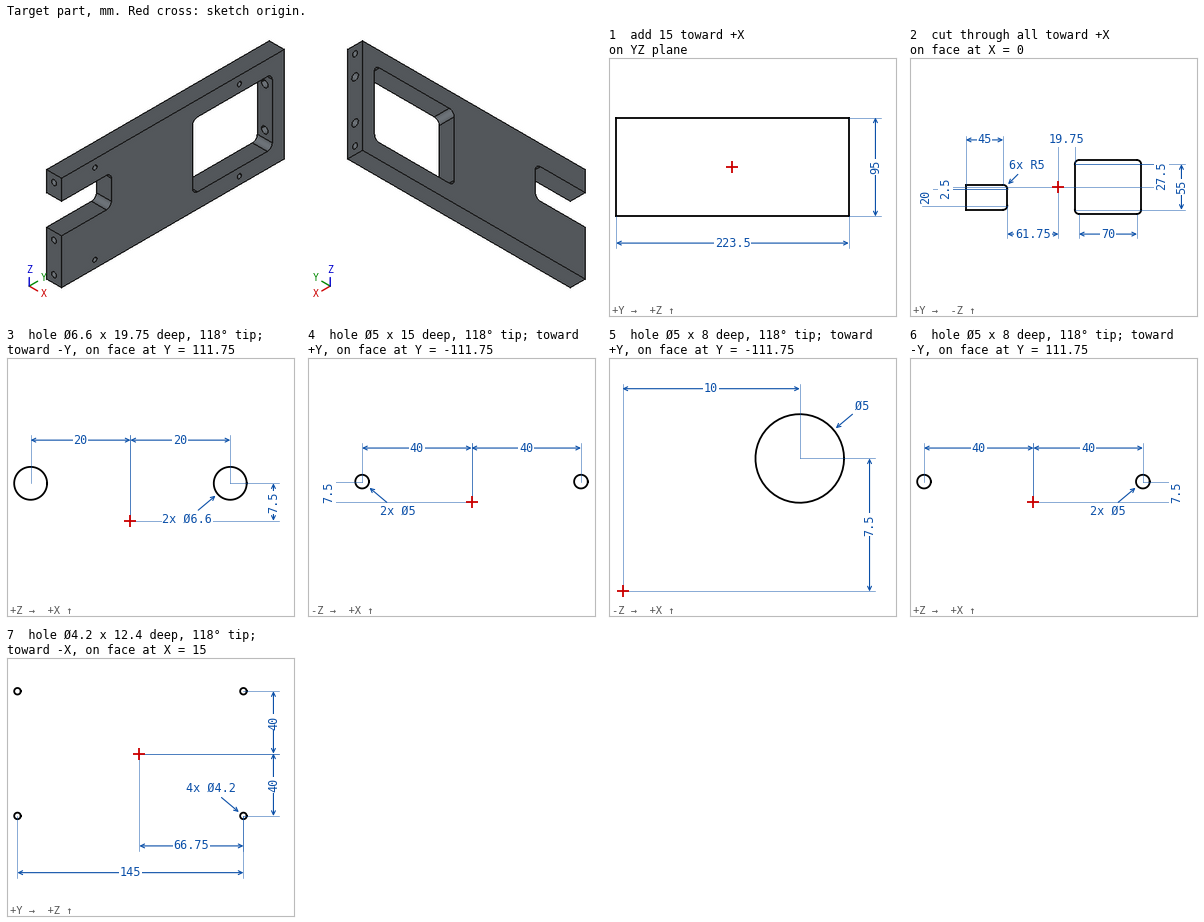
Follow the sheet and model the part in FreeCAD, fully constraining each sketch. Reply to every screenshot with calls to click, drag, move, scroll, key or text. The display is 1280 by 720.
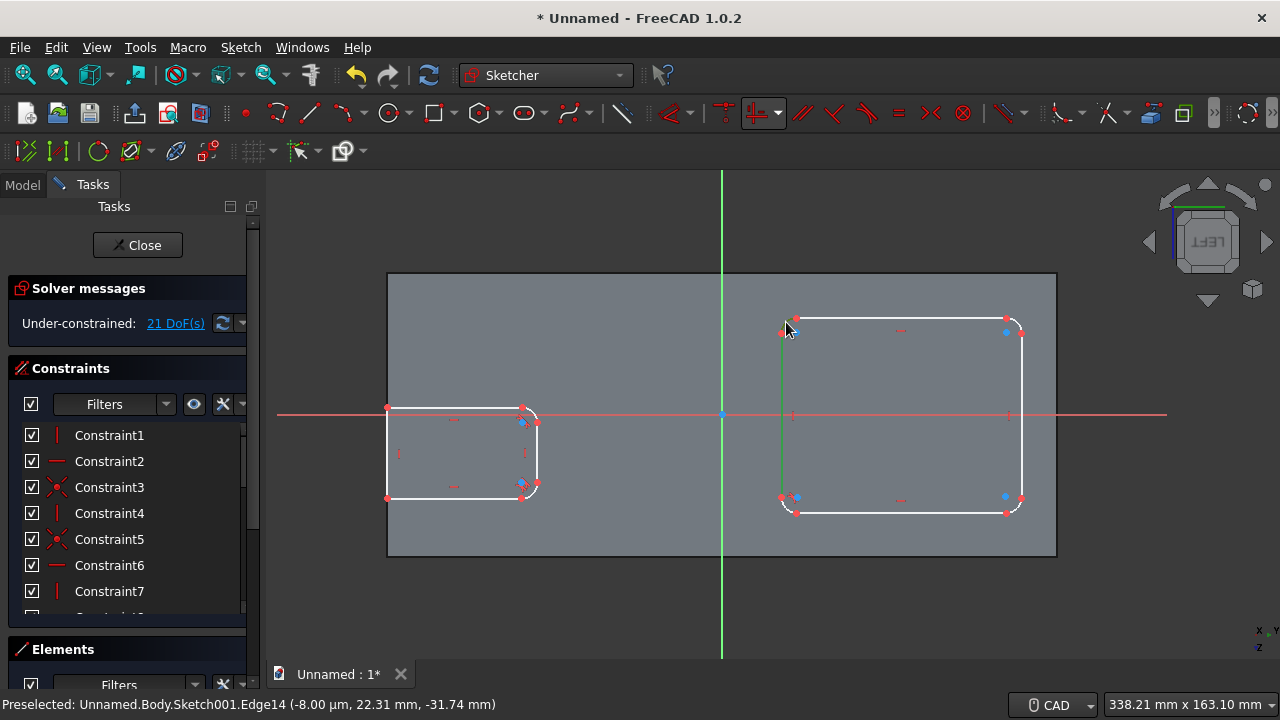
click(868, 114)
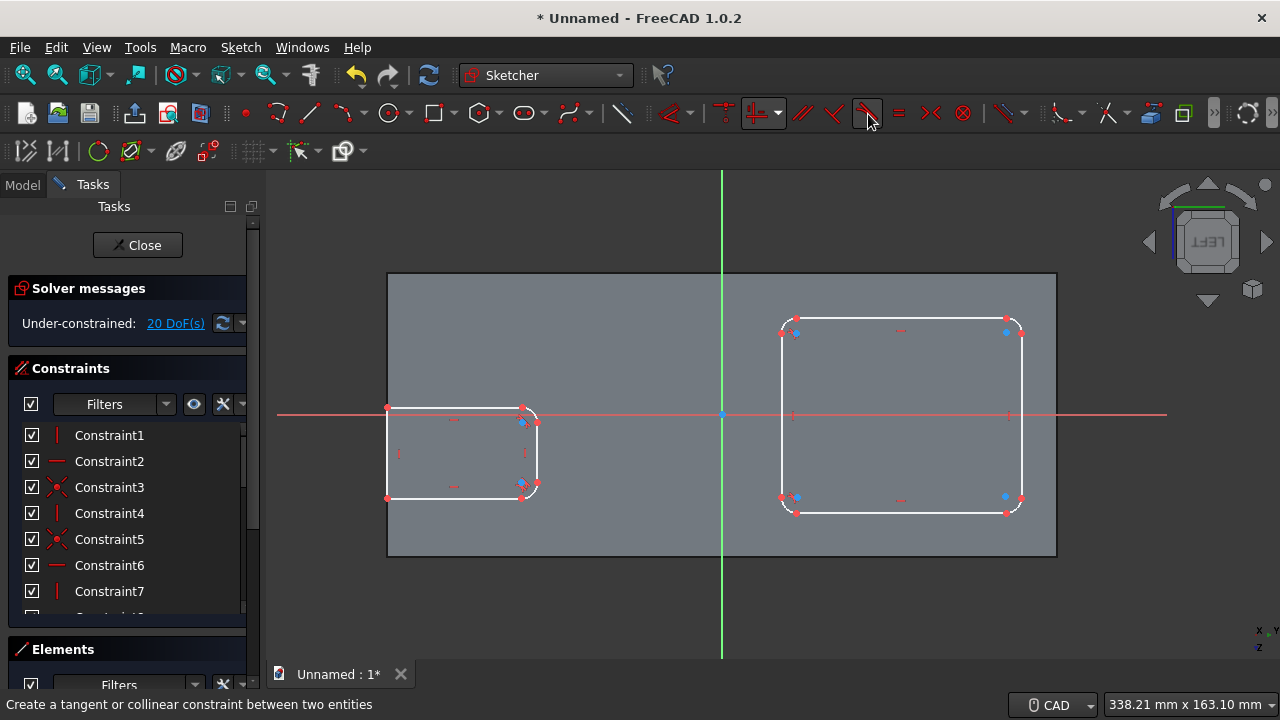
click(860, 513)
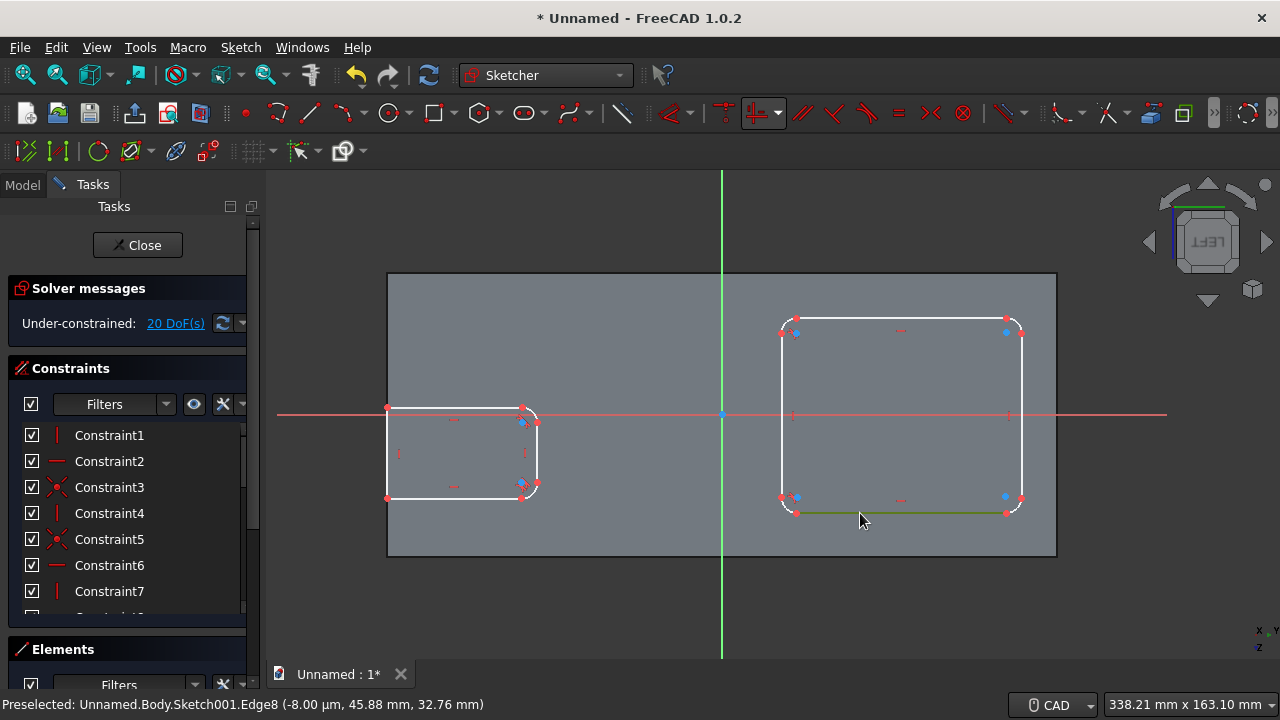
click(786, 508)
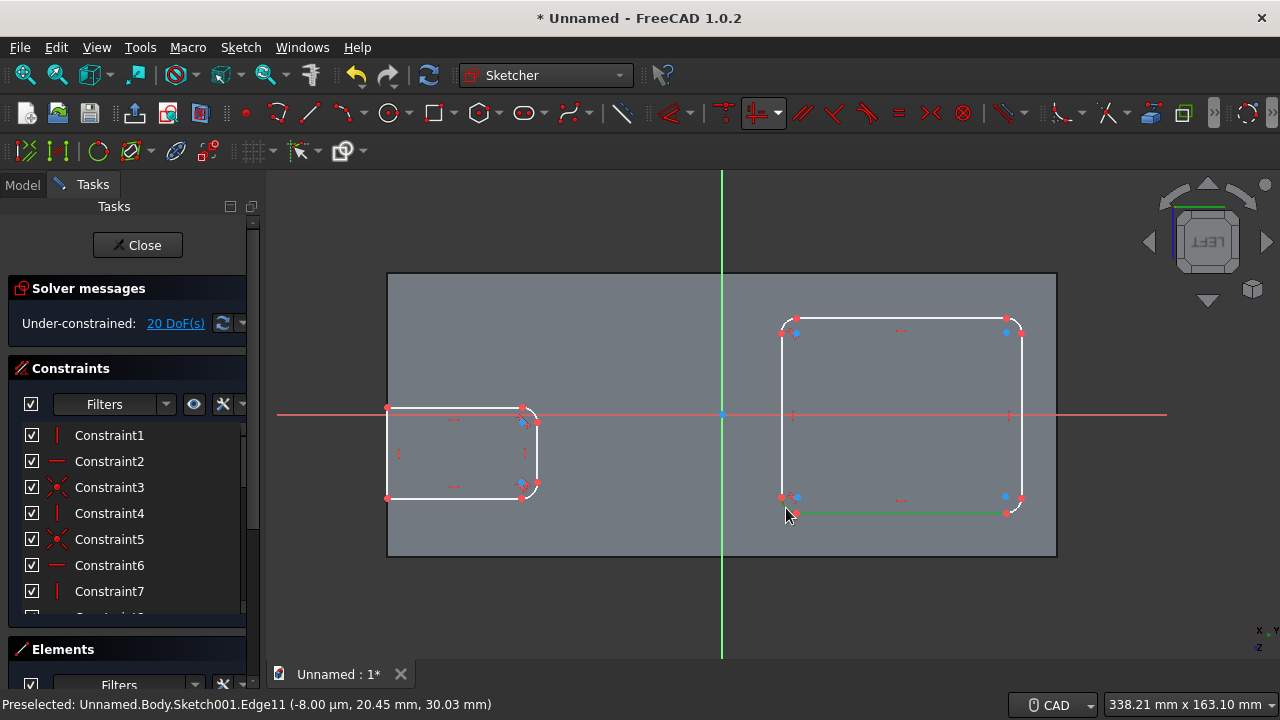
key(t)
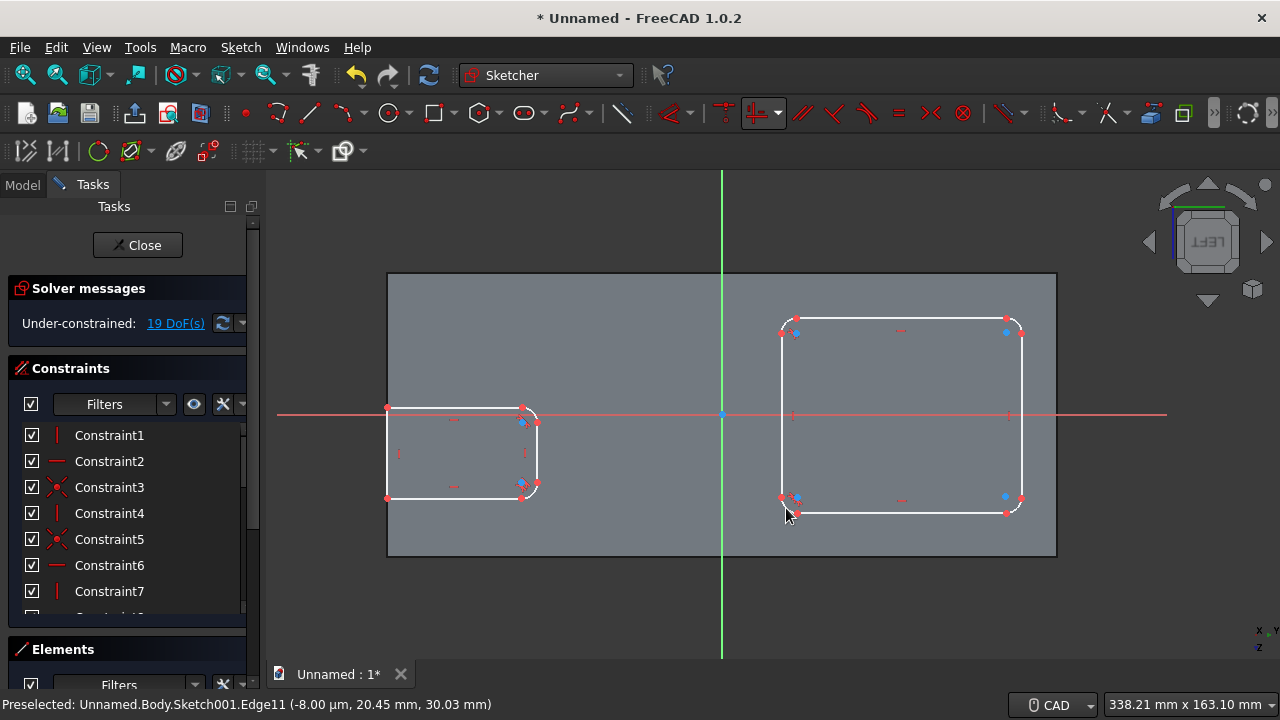
click(860, 513)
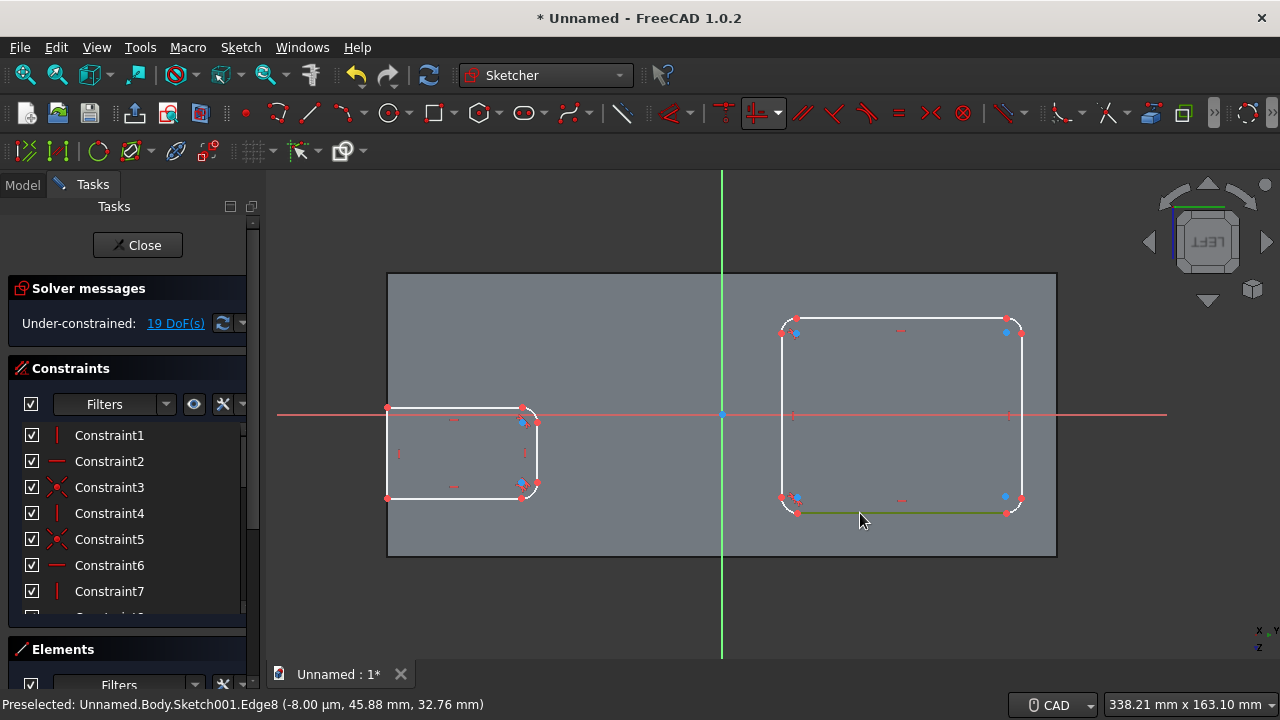
scroll(1017, 508, up, 2)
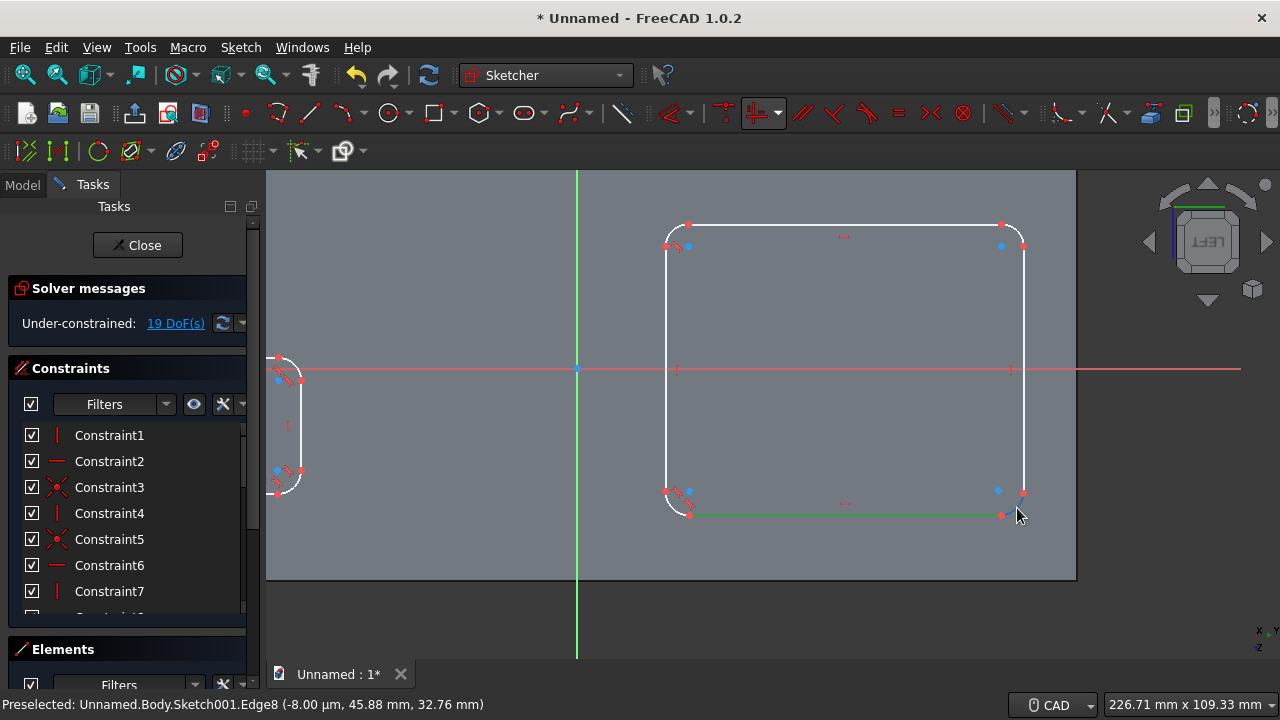
click(1016, 508)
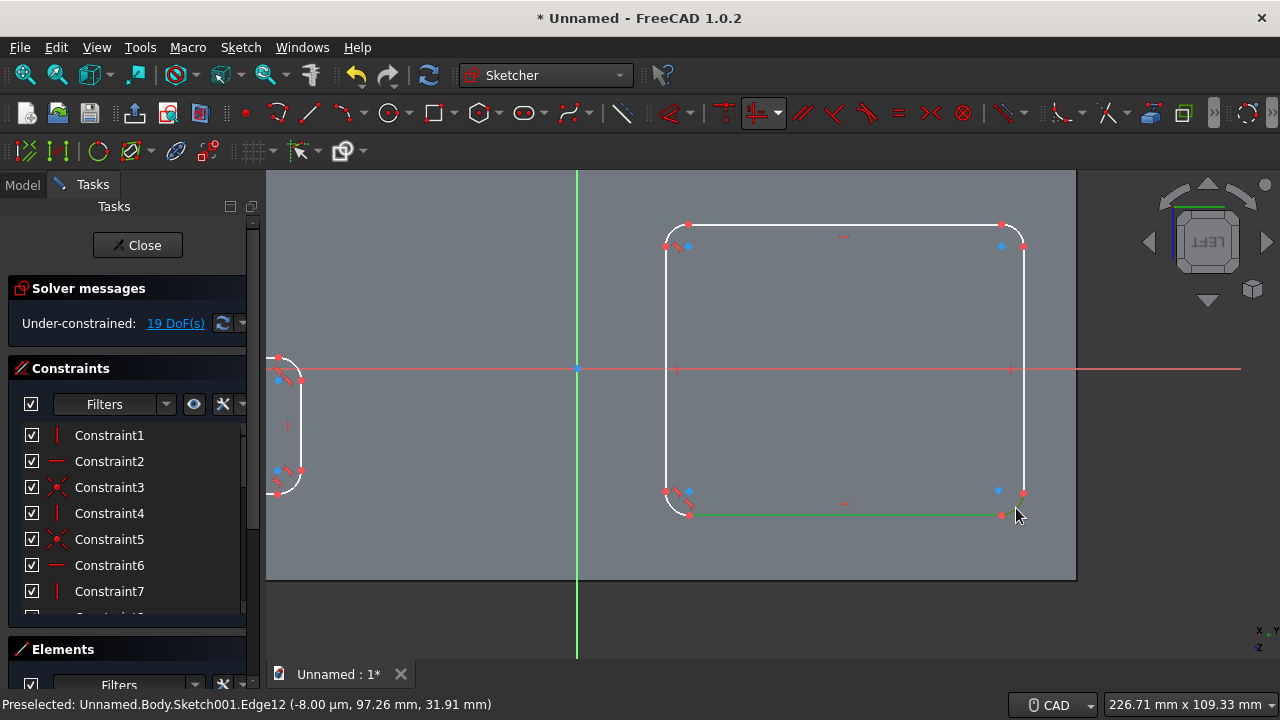
click(868, 114)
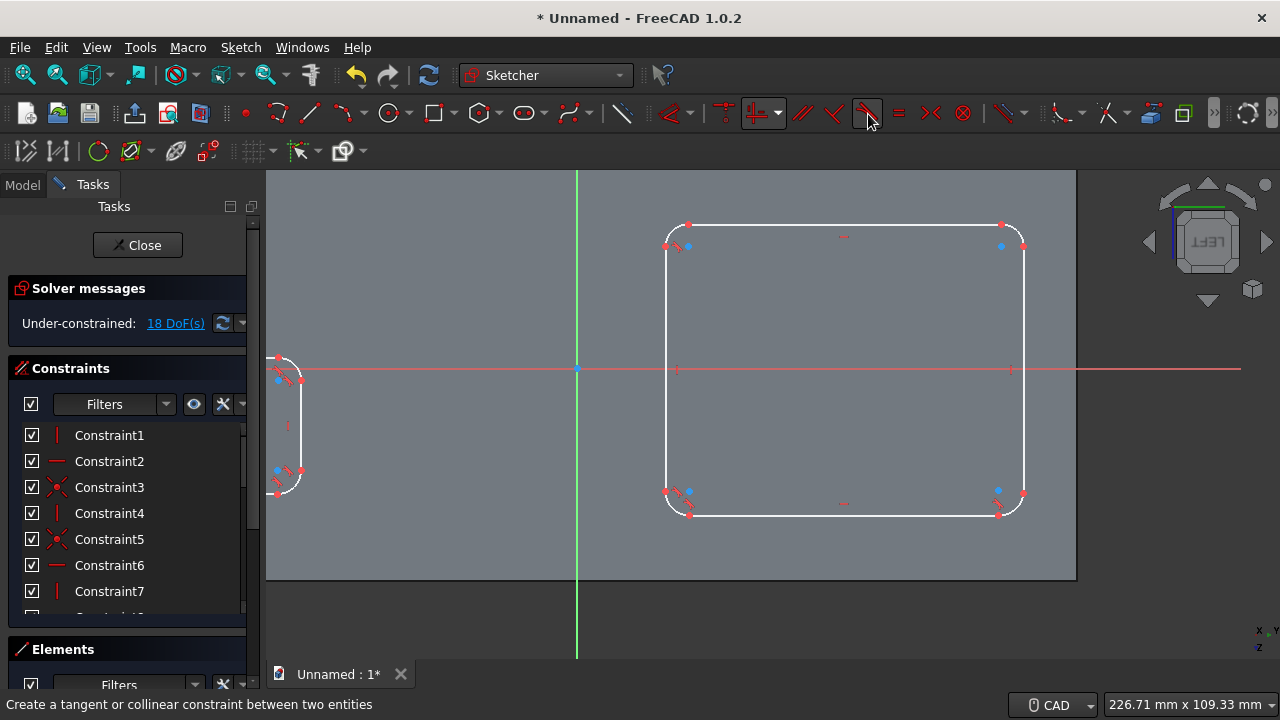
click(1024, 419)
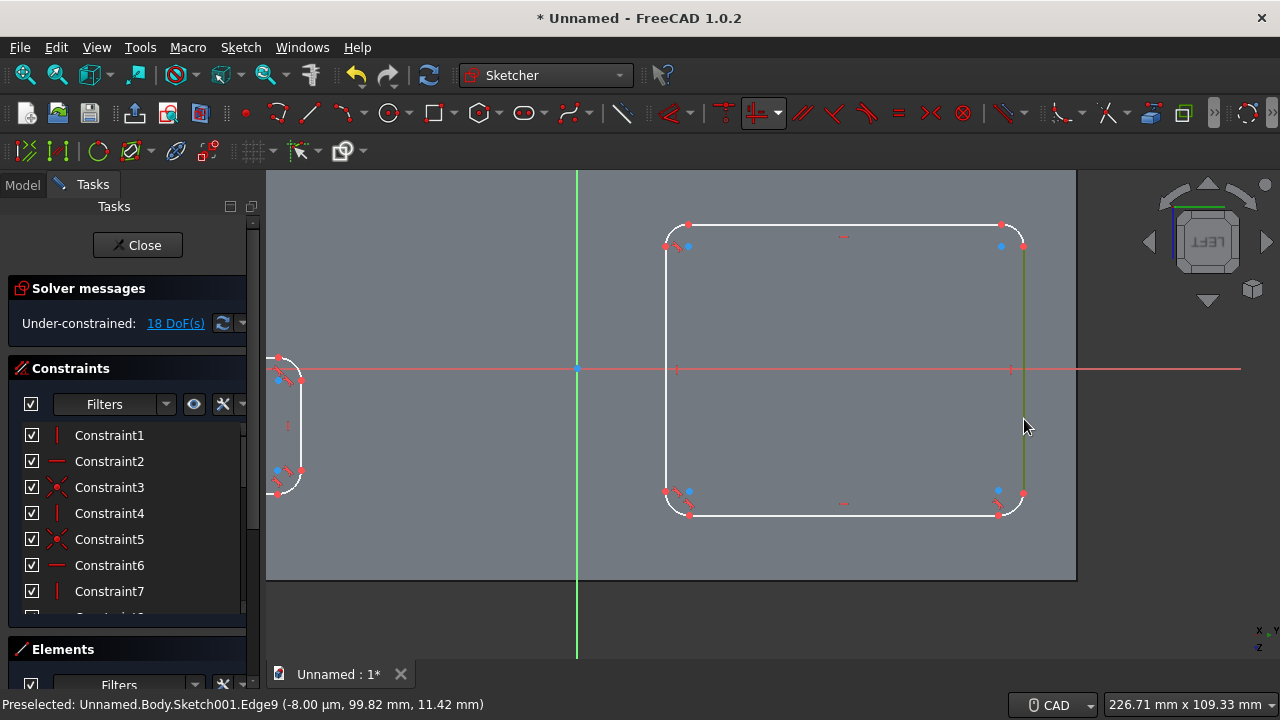
scroll(1009, 513, up, 2)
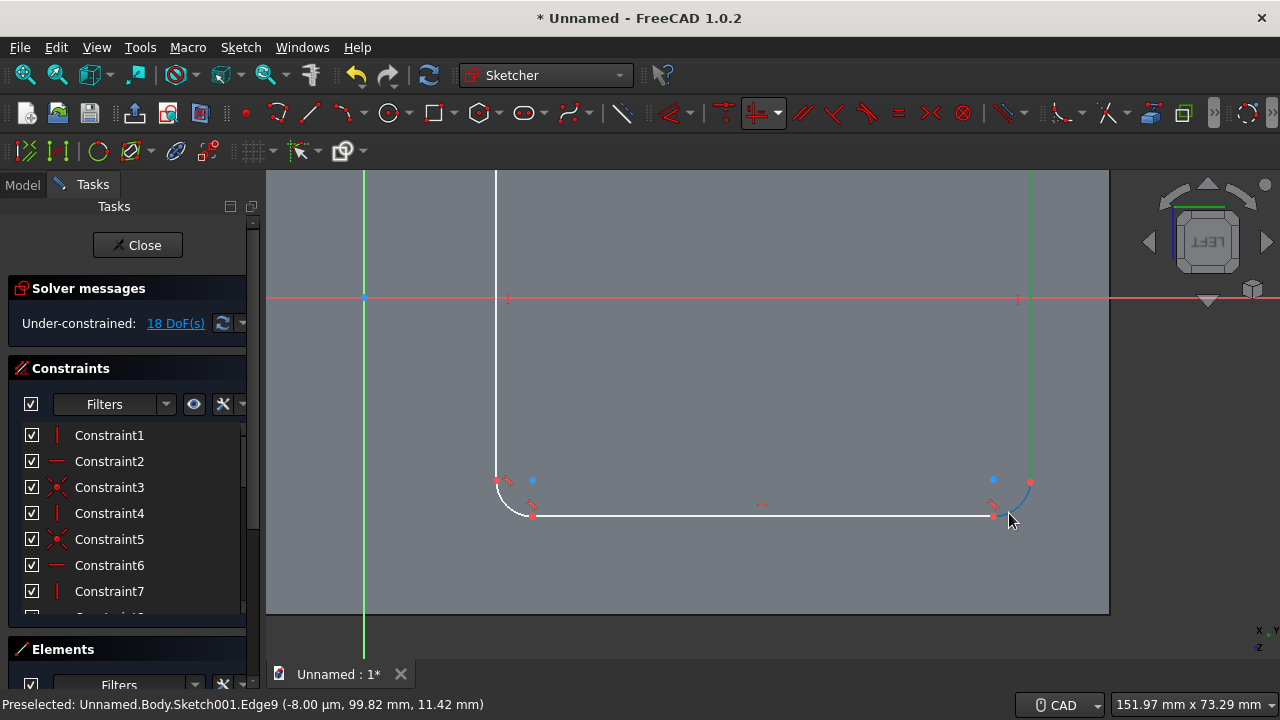
click(1009, 513)